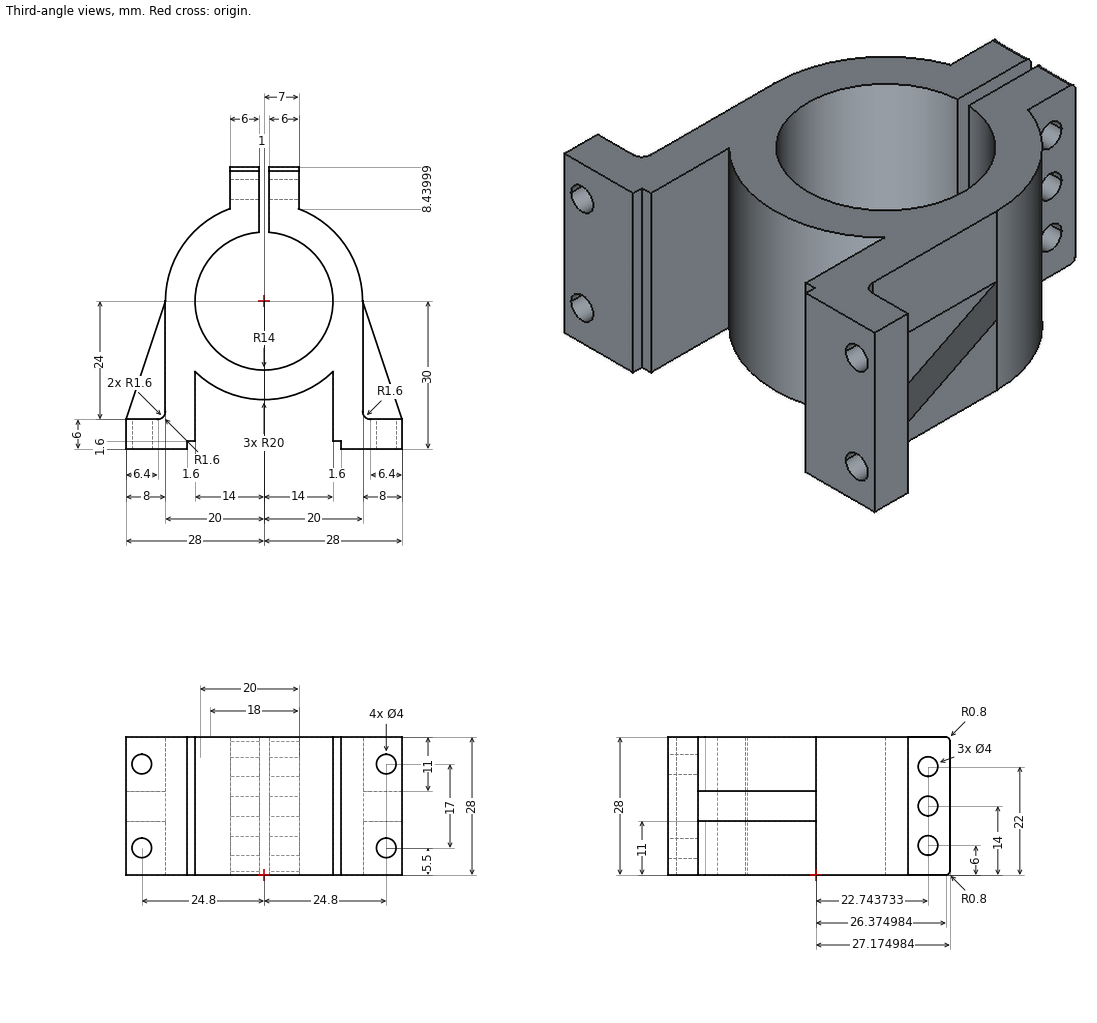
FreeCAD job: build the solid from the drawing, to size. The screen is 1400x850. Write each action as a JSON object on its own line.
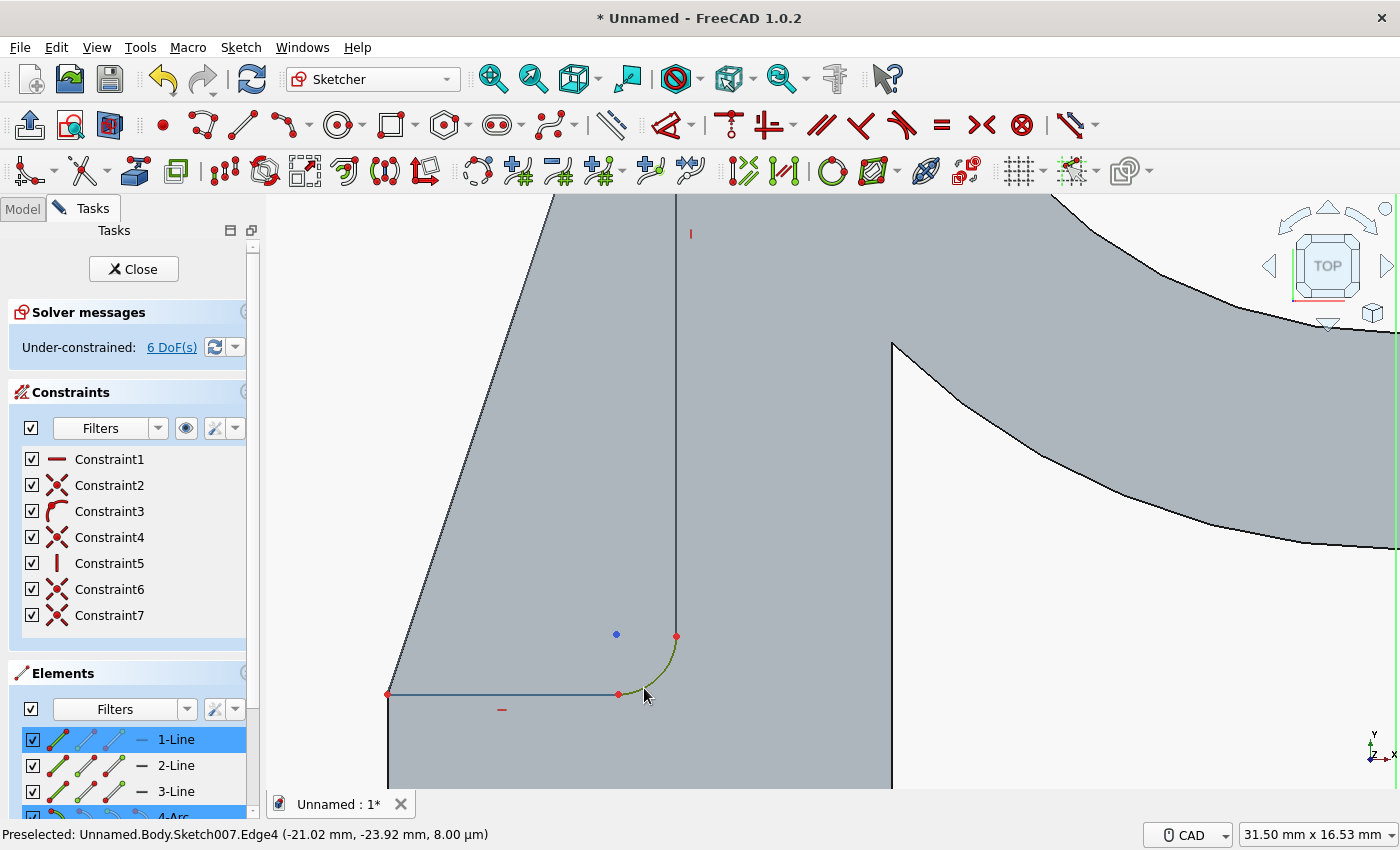
{"action": "left_click", "coordinate": [902, 126]}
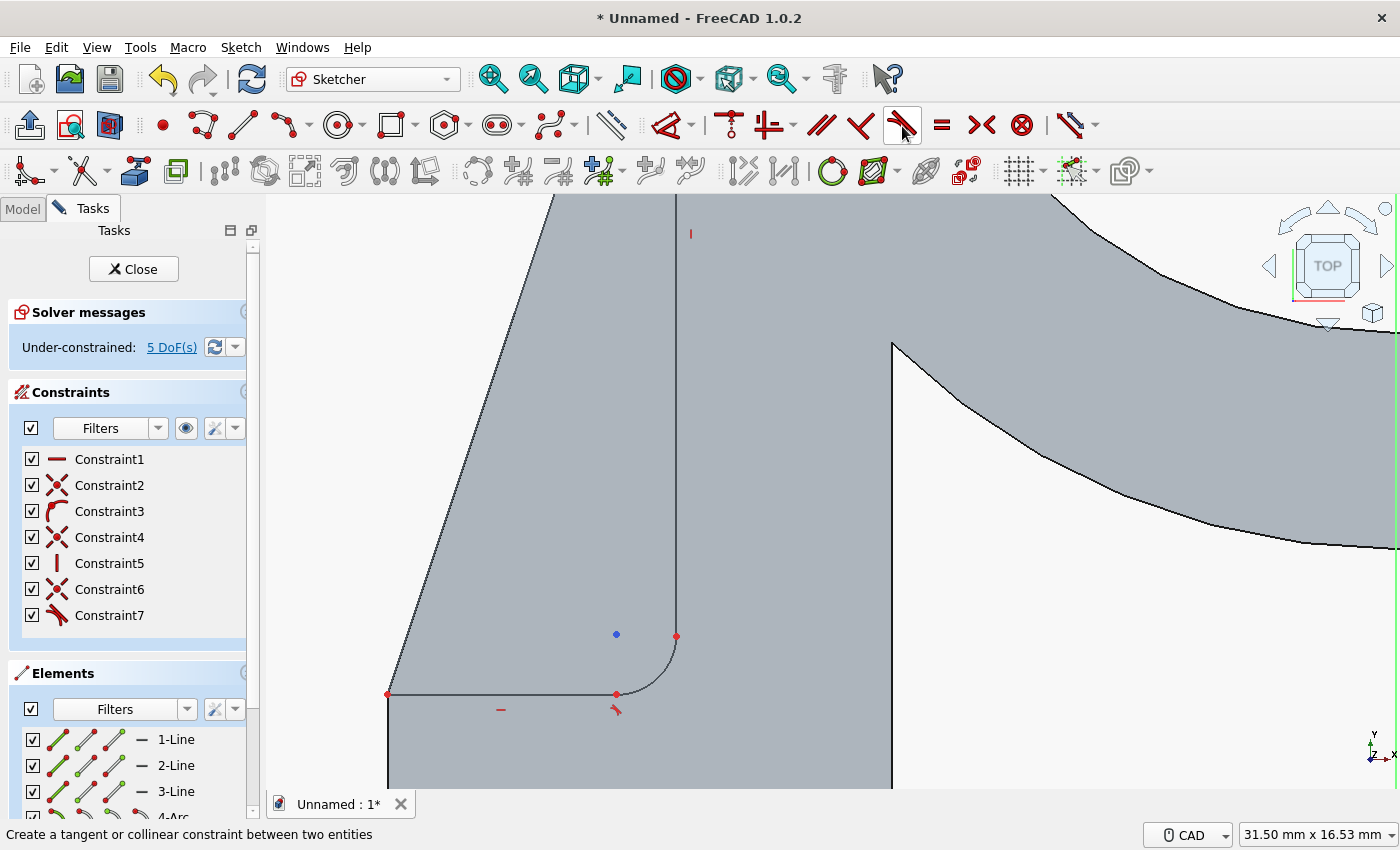
{"action": "left_click", "coordinate": [676, 395]}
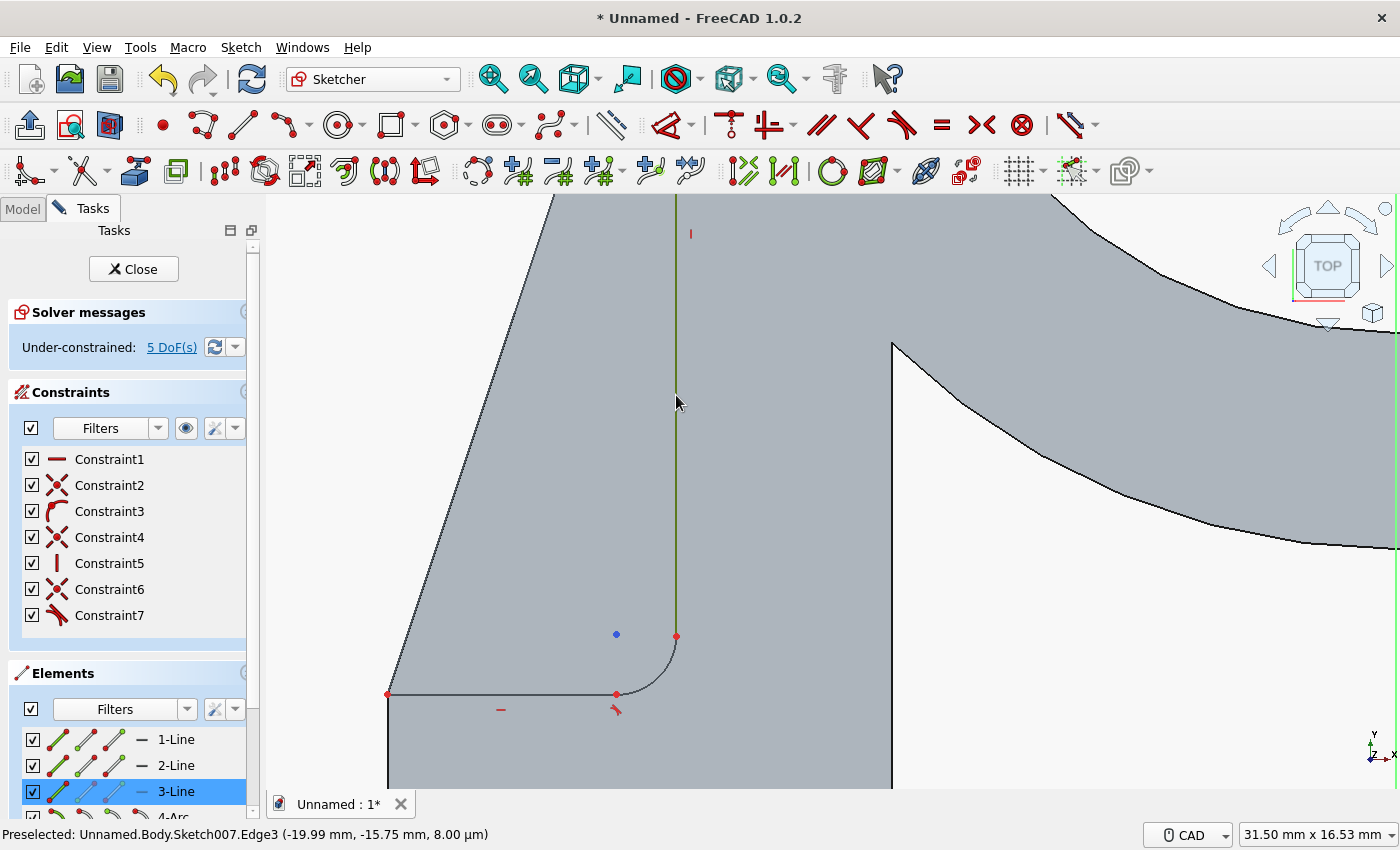
{"action": "left_click", "coordinate": [643, 689]}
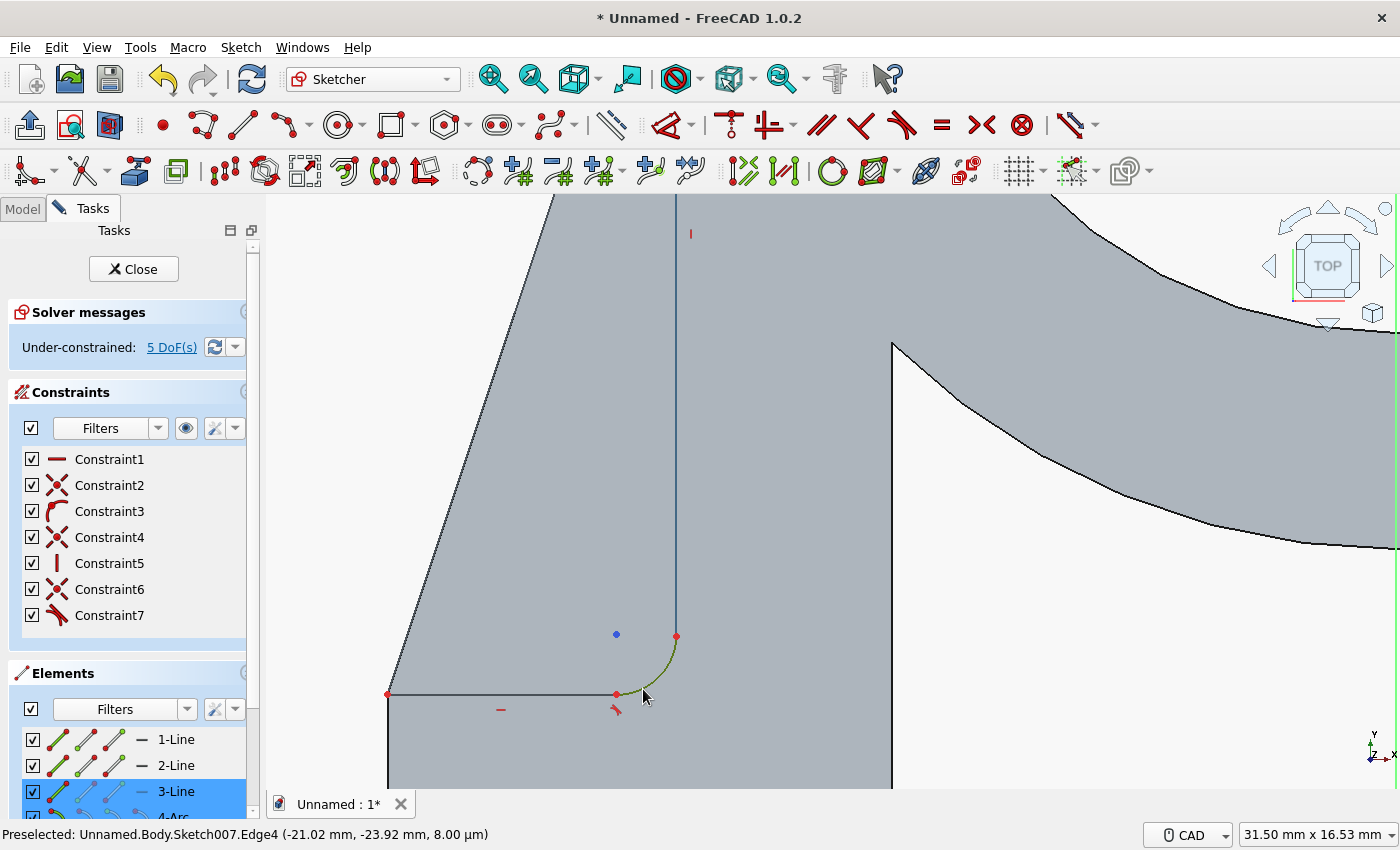
{"action": "left_click", "coordinate": [902, 126]}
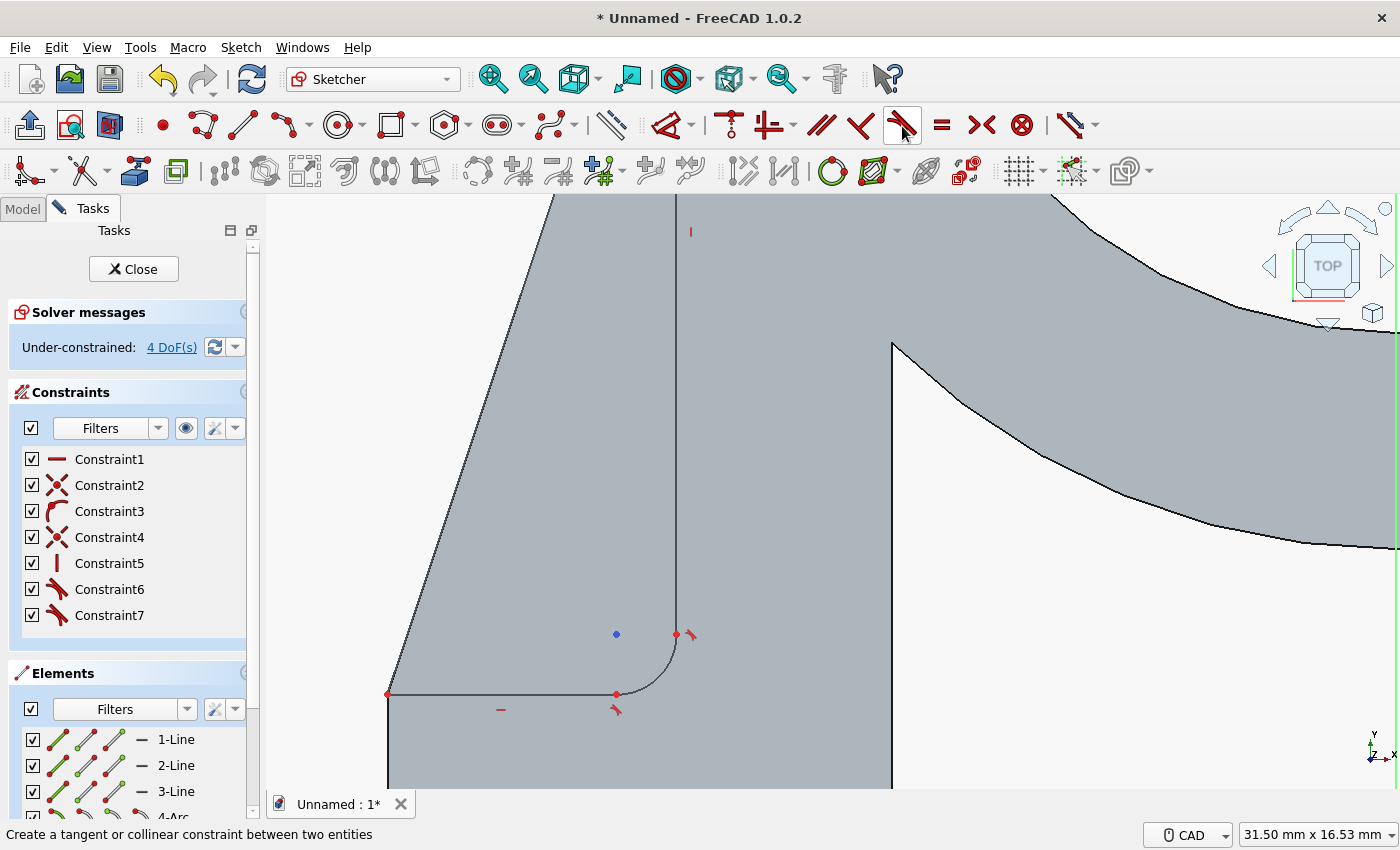
{"action": "left_click", "coordinate": [666, 126]}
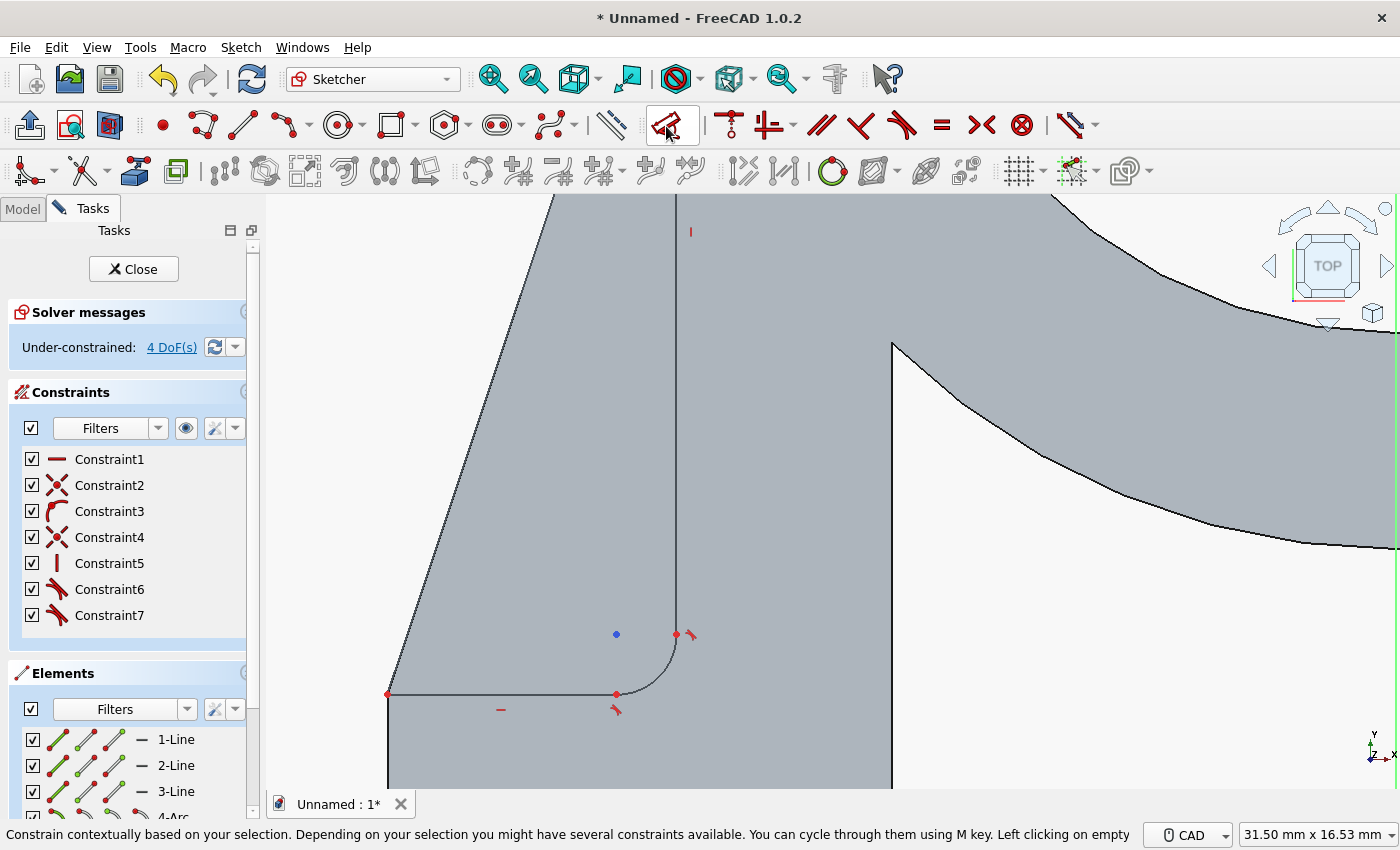
{"action": "left_click", "coordinate": [644, 688]}
{"action": "left_click", "coordinate": [659, 716]}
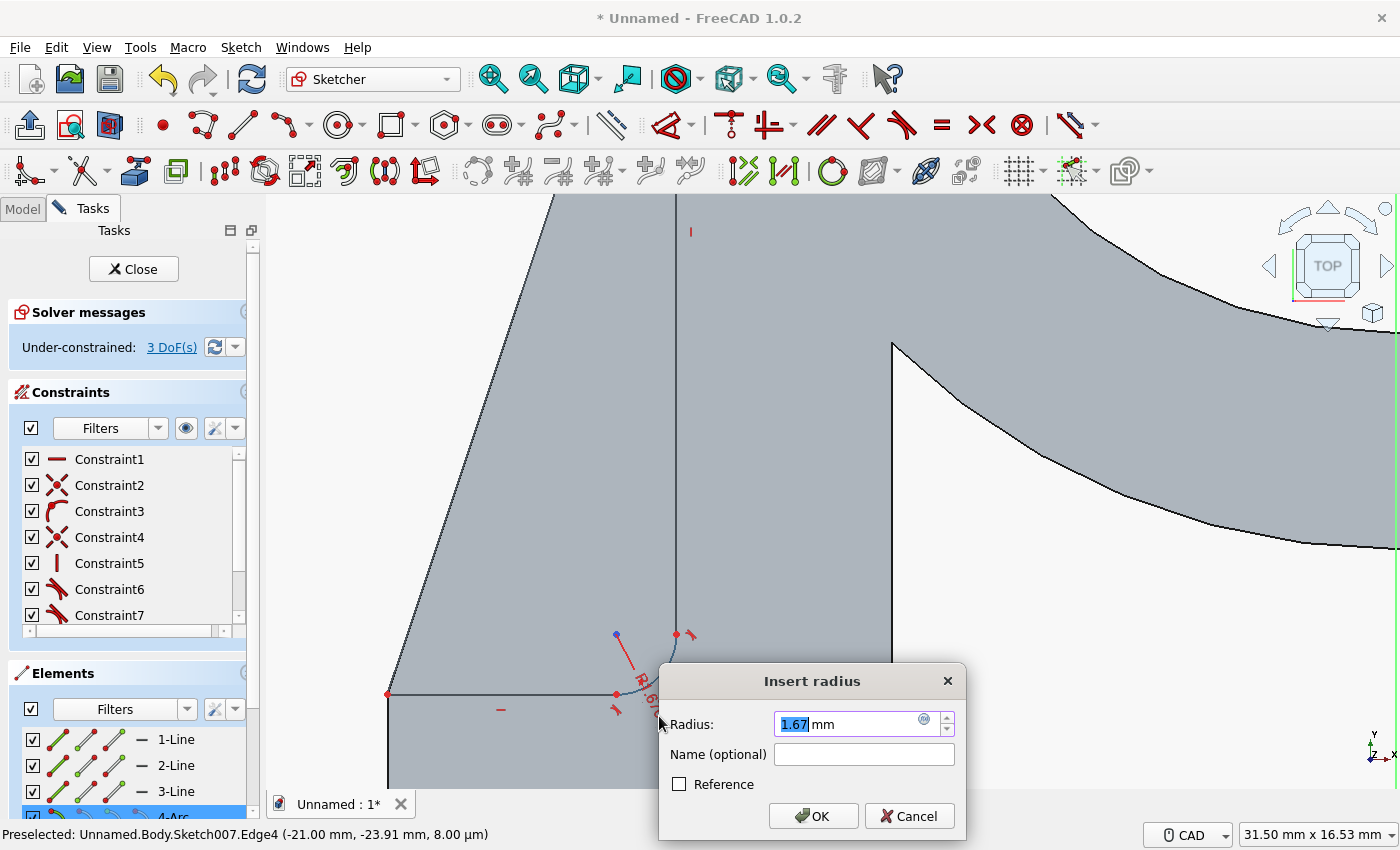
{"action": "type", "text": "1.6"}
{"action": "key", "text": "Return"}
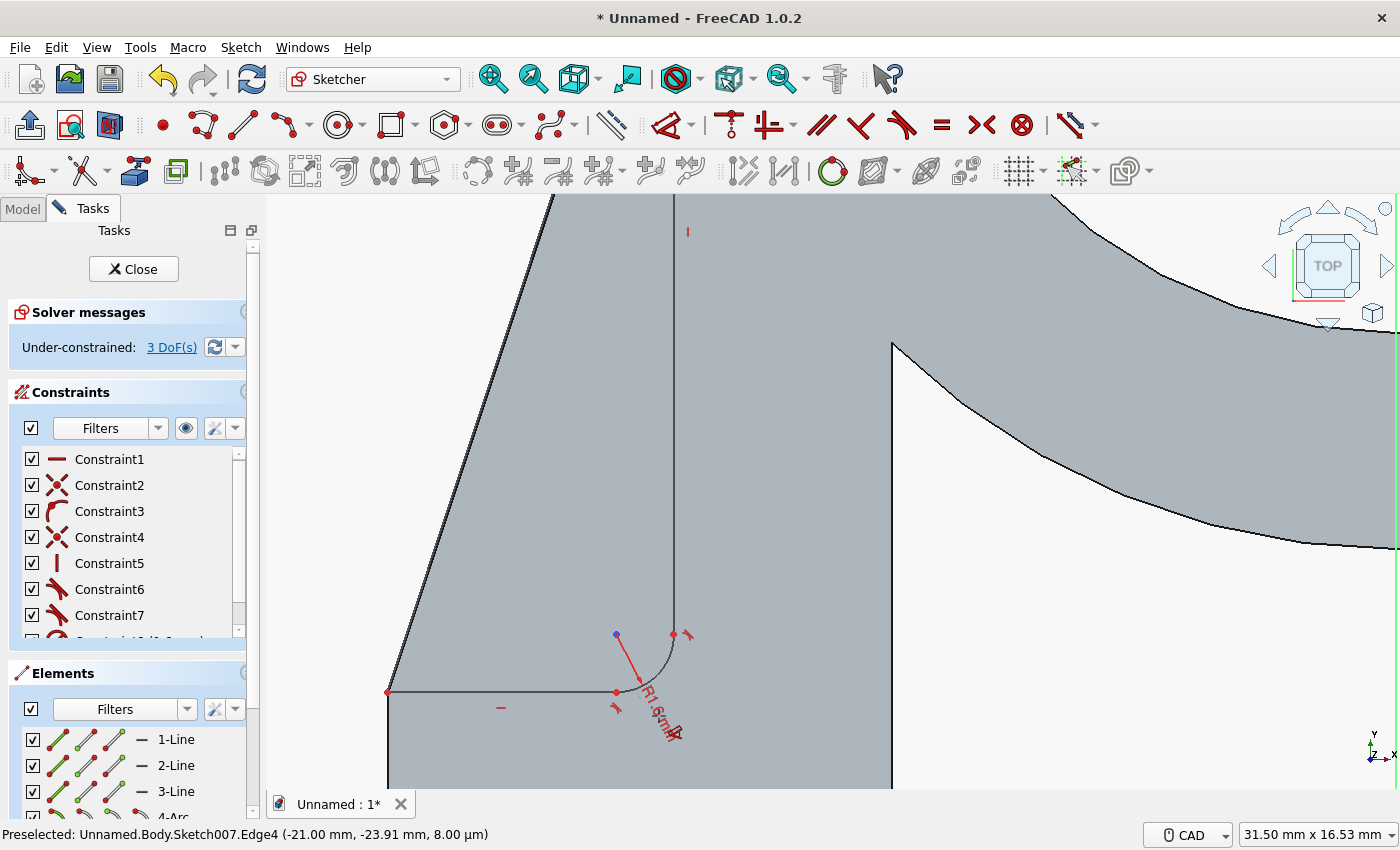
{"action": "left_click", "coordinate": [473, 433]}
{"action": "left_click", "coordinate": [530, 726]}